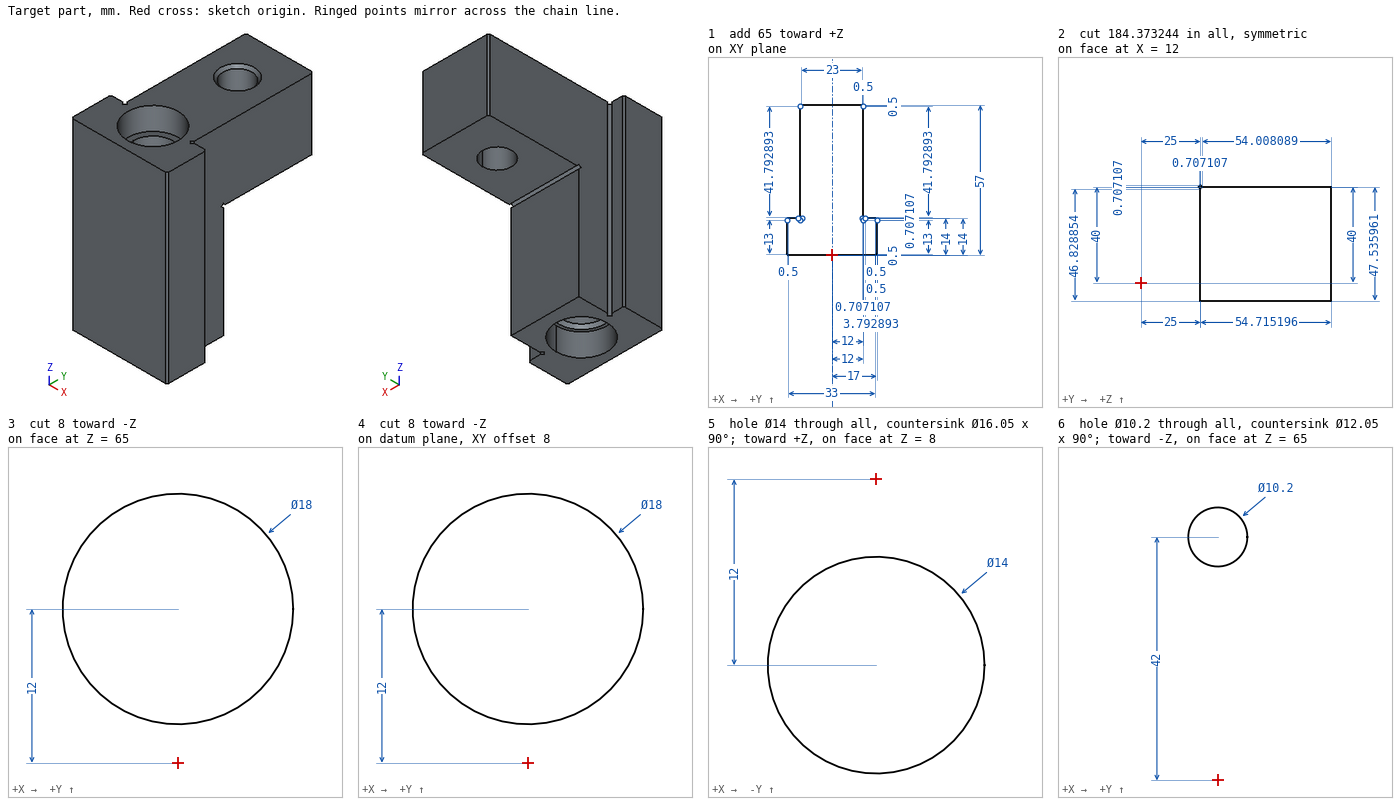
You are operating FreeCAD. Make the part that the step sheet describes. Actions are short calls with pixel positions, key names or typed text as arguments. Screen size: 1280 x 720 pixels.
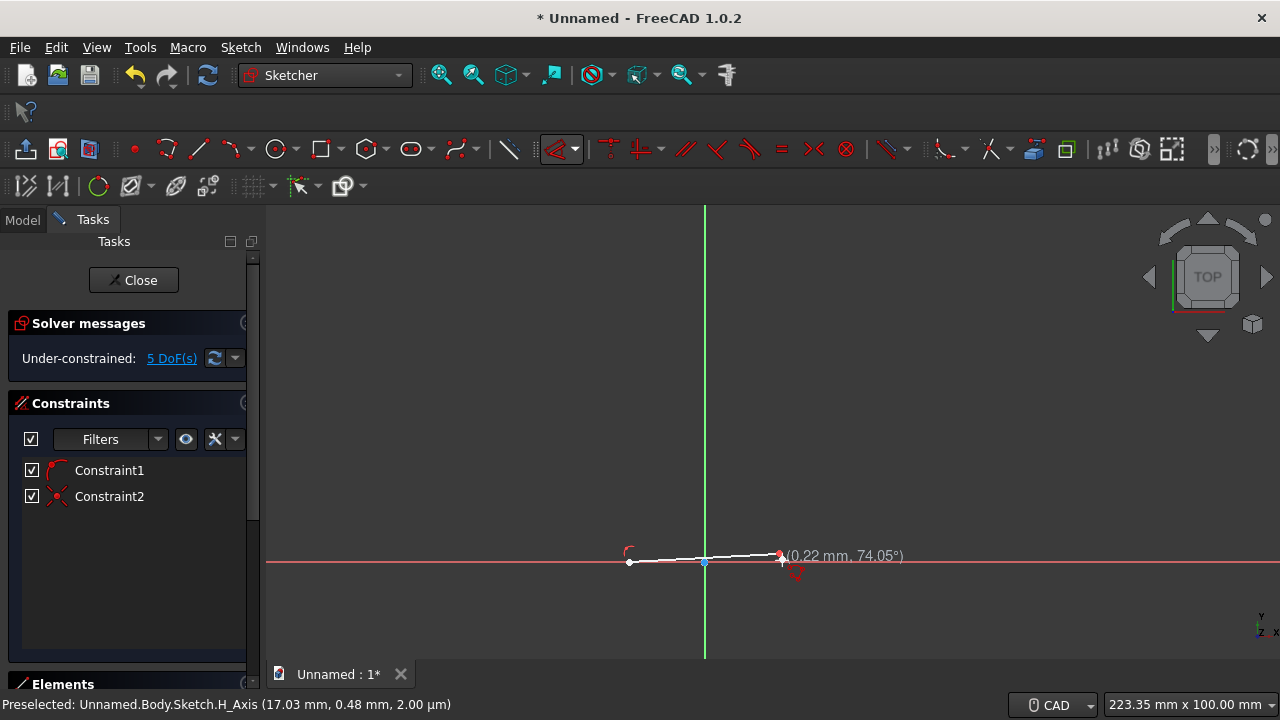
click(782, 501)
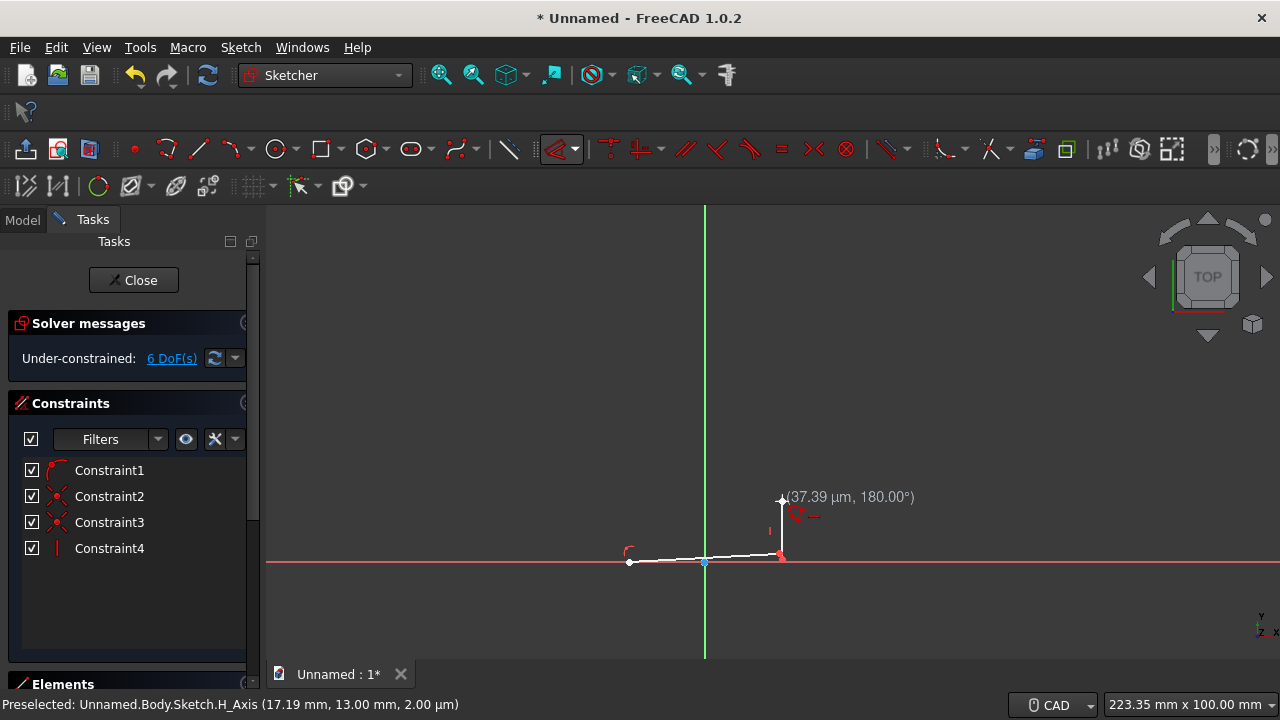
scroll(780, 498, up, 8)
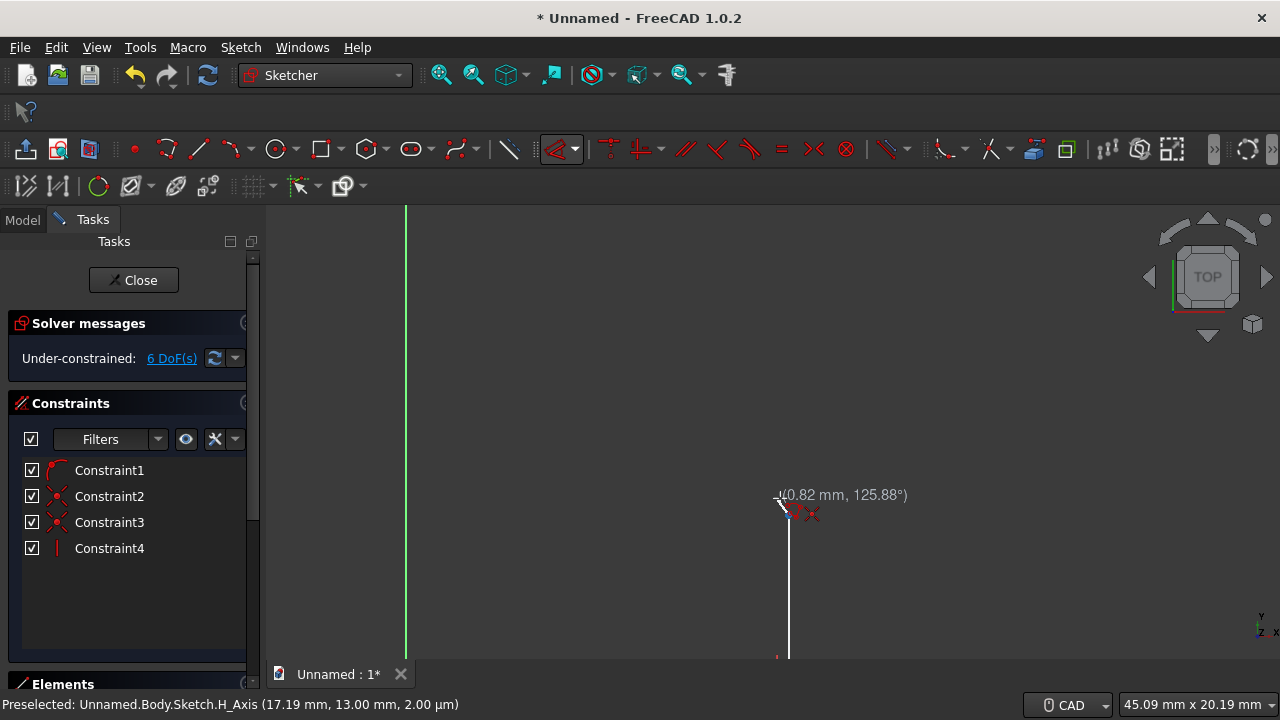
click(777, 498)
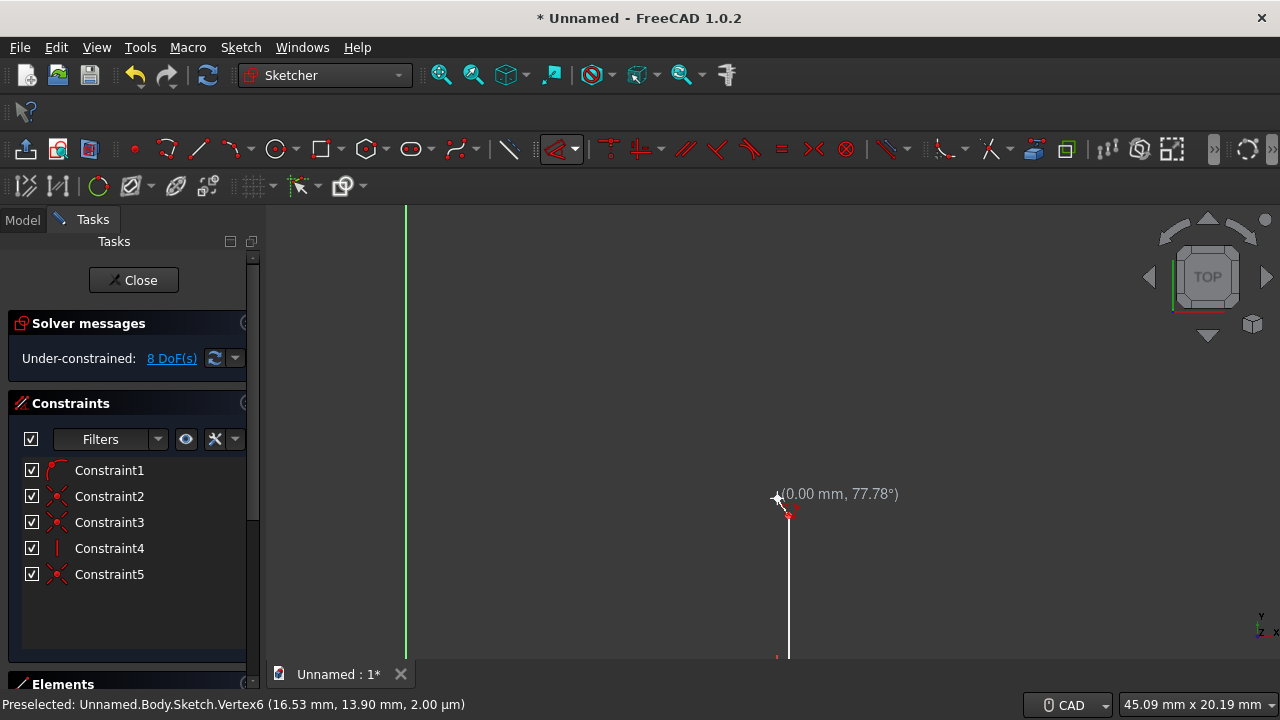
scroll(780, 498, down, 8)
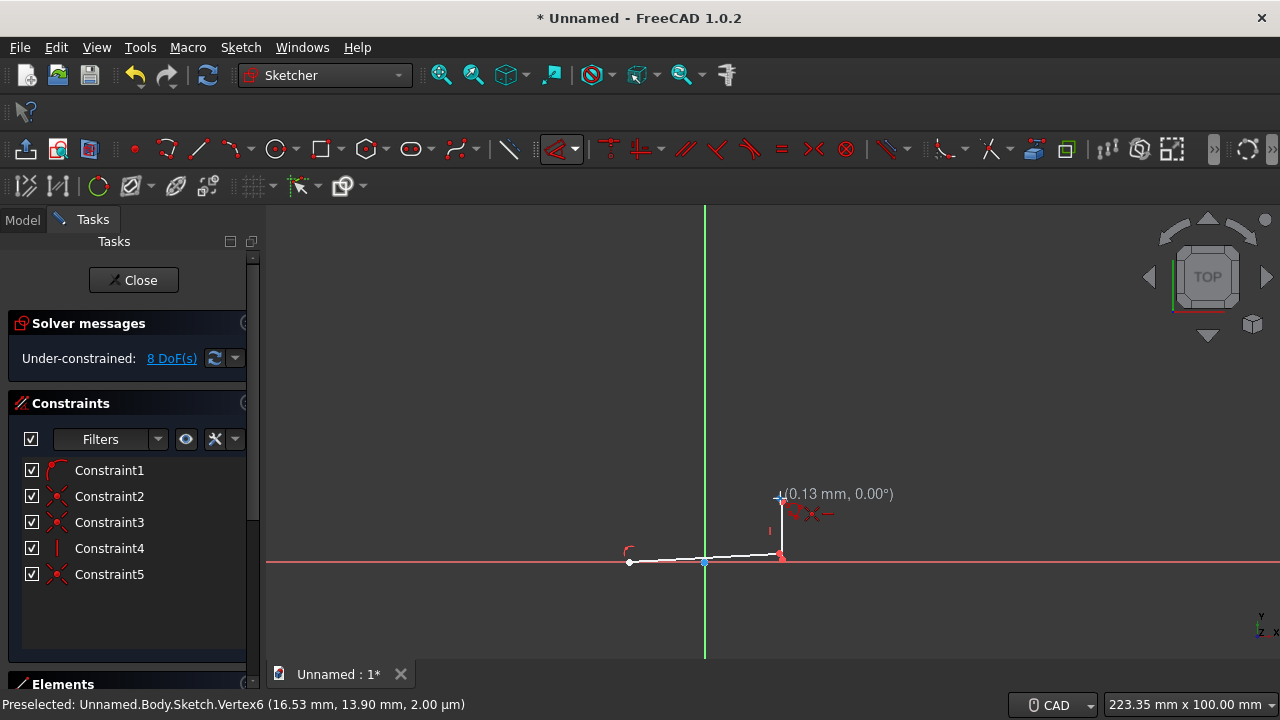
click(763, 499)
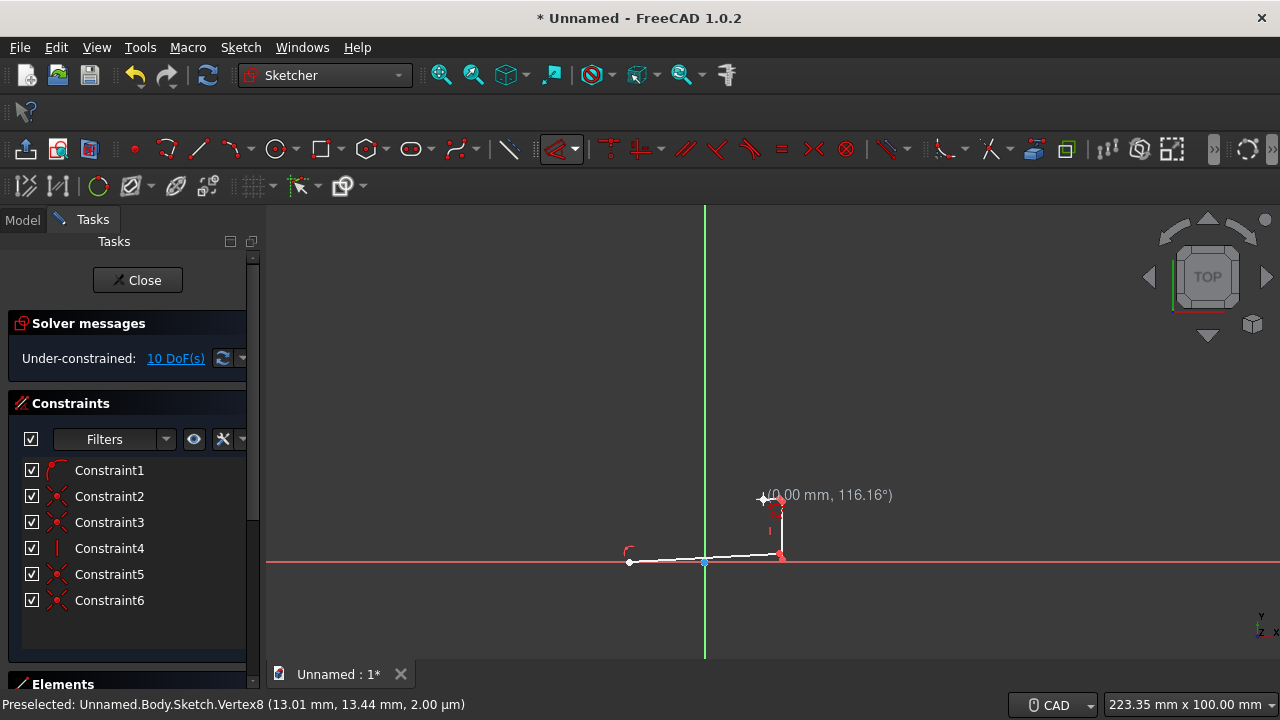
scroll(759, 502, up, 7)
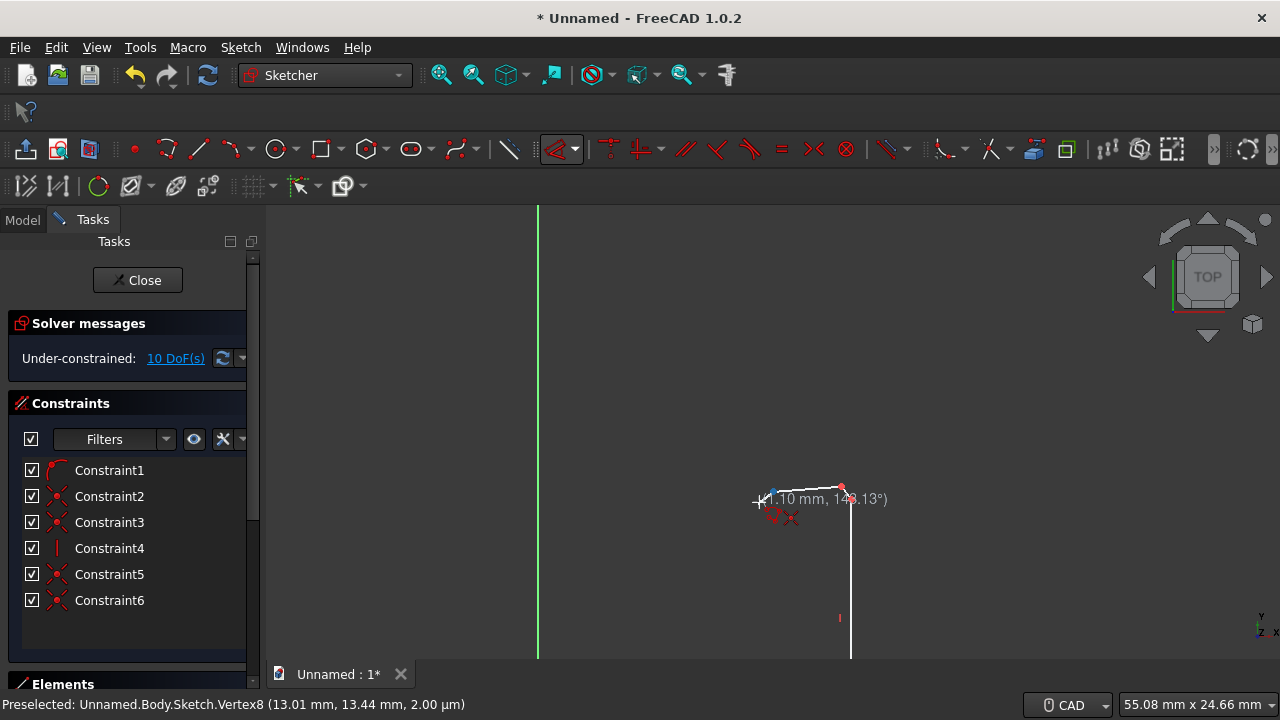
click(759, 499)
click(746, 486)
click(759, 473)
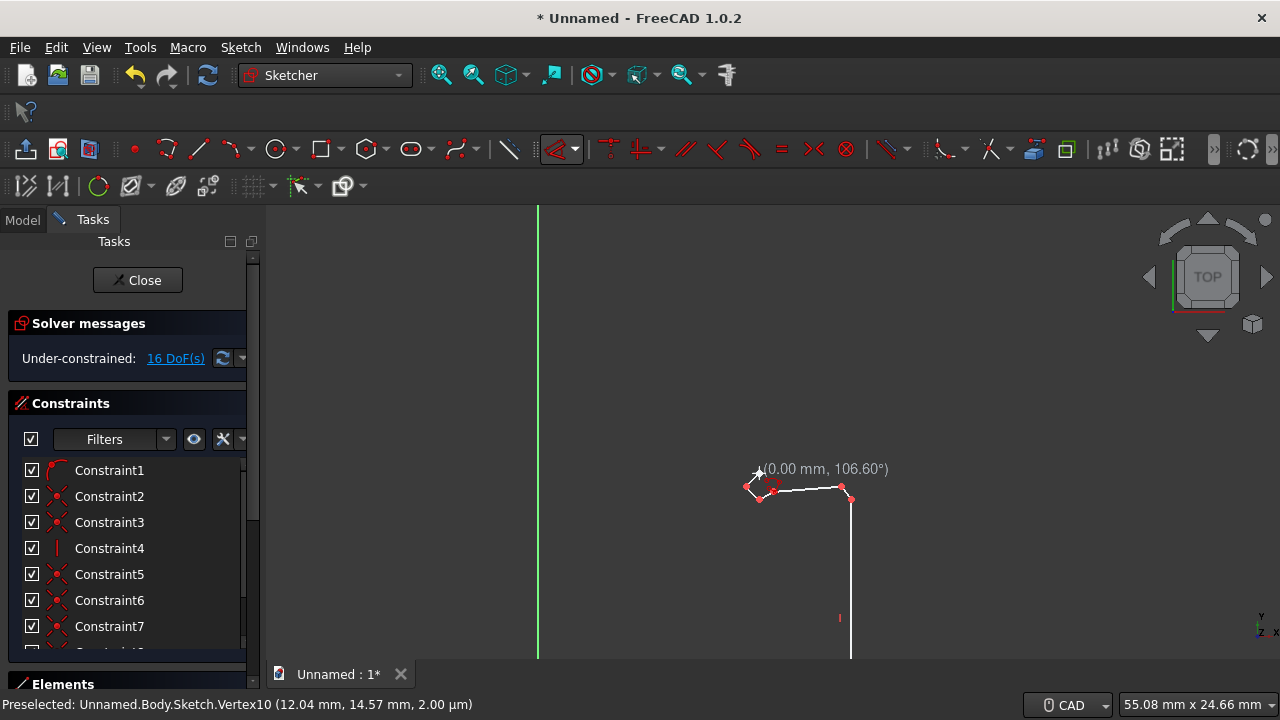
scroll(759, 502, down, 7)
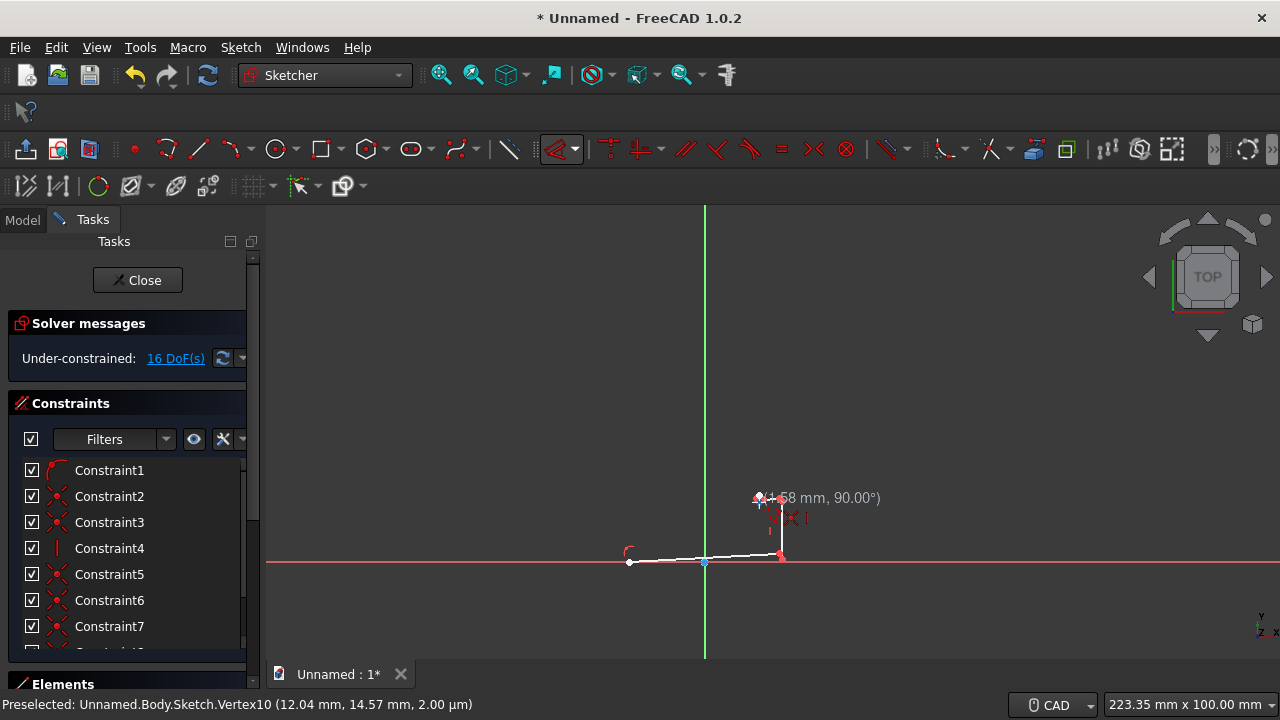
click(759, 305)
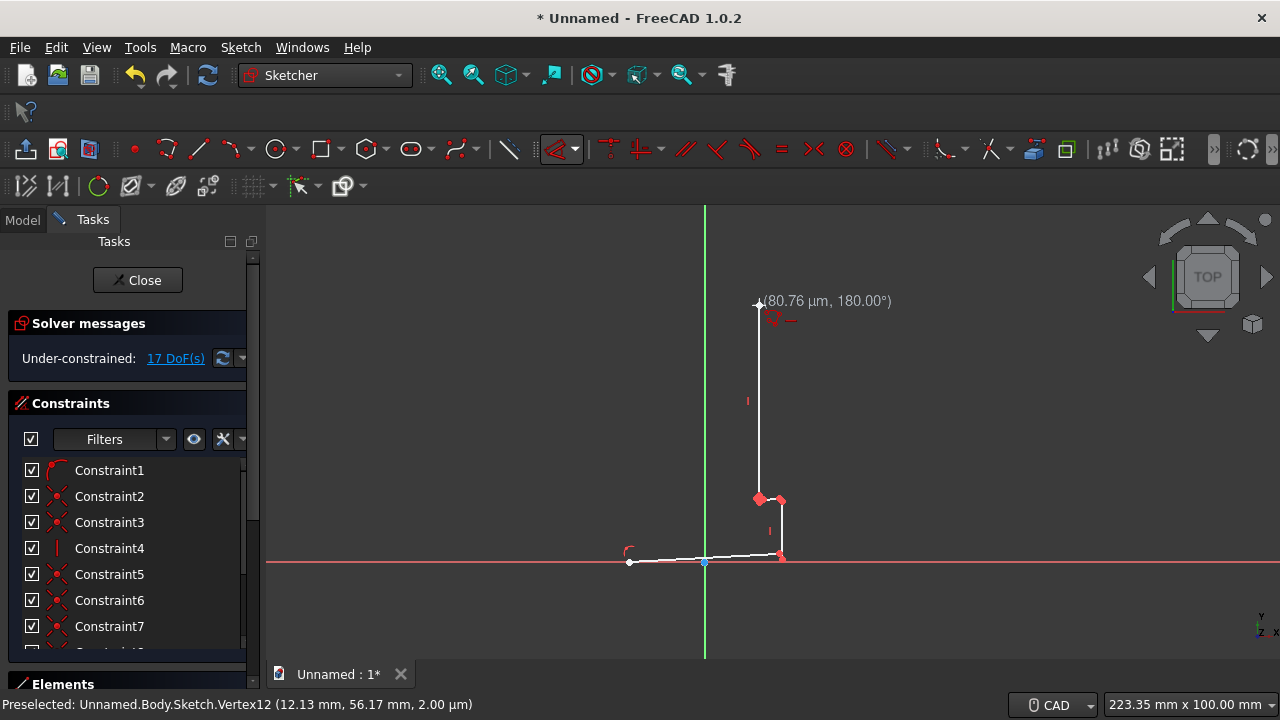
scroll(757, 303, up, 8)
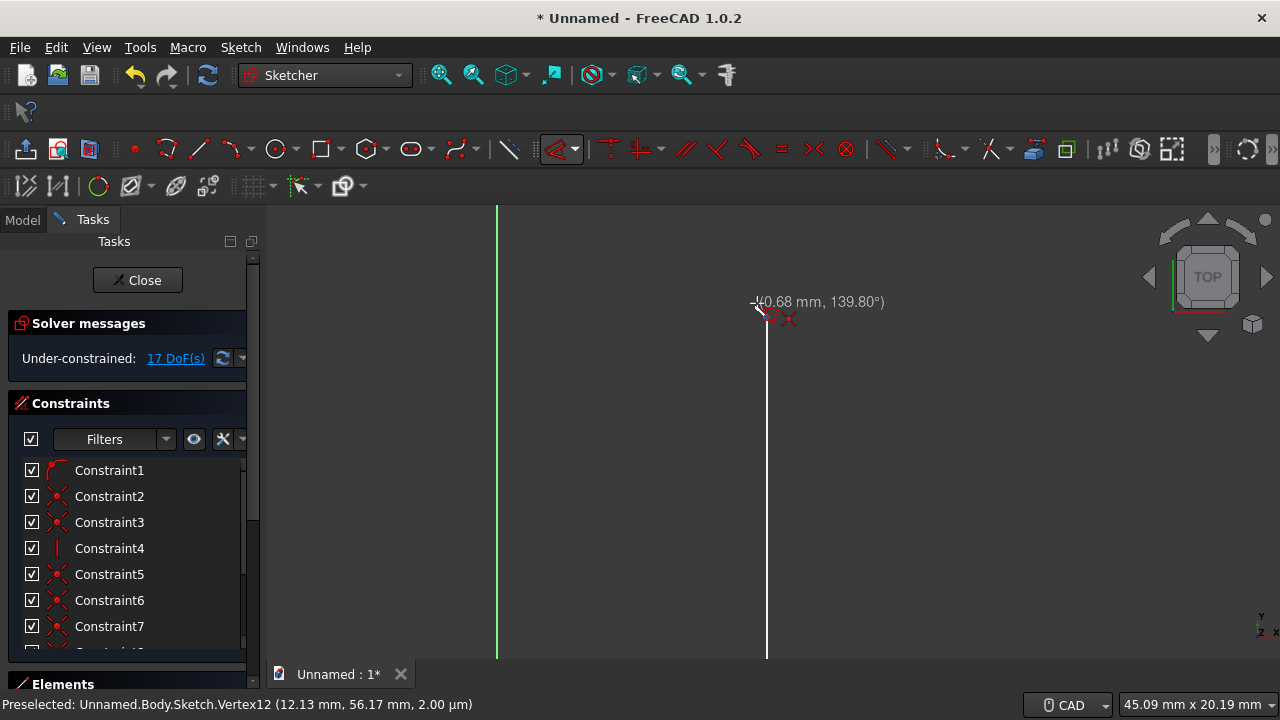
click(756, 303)